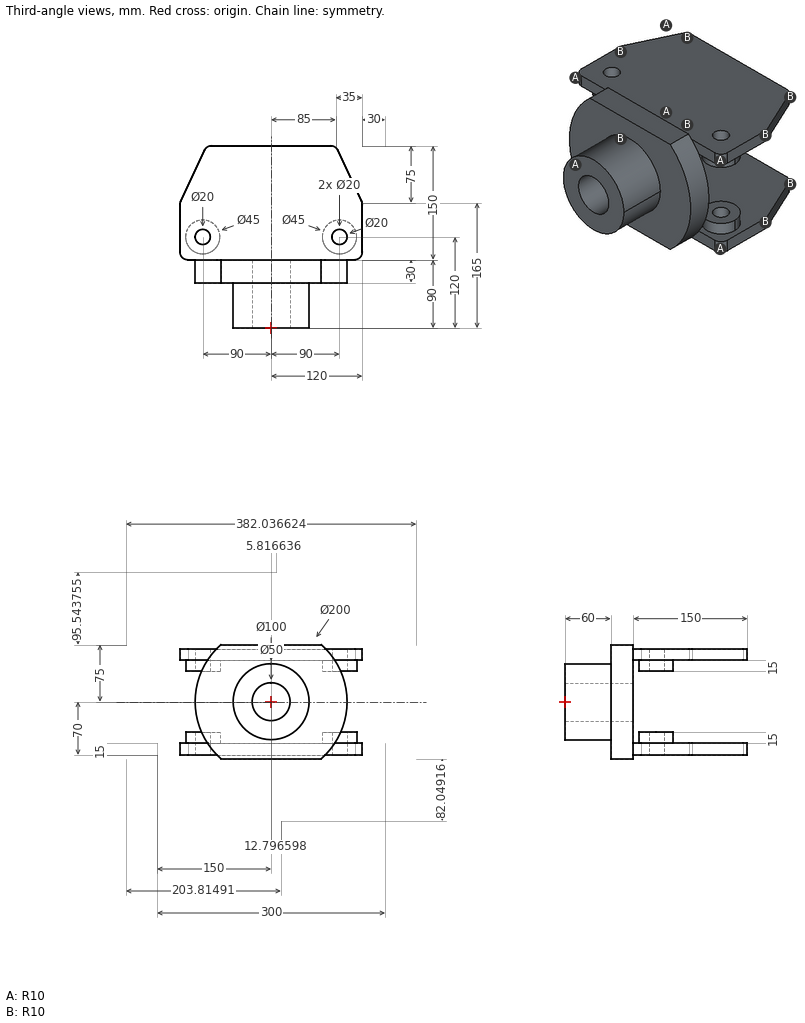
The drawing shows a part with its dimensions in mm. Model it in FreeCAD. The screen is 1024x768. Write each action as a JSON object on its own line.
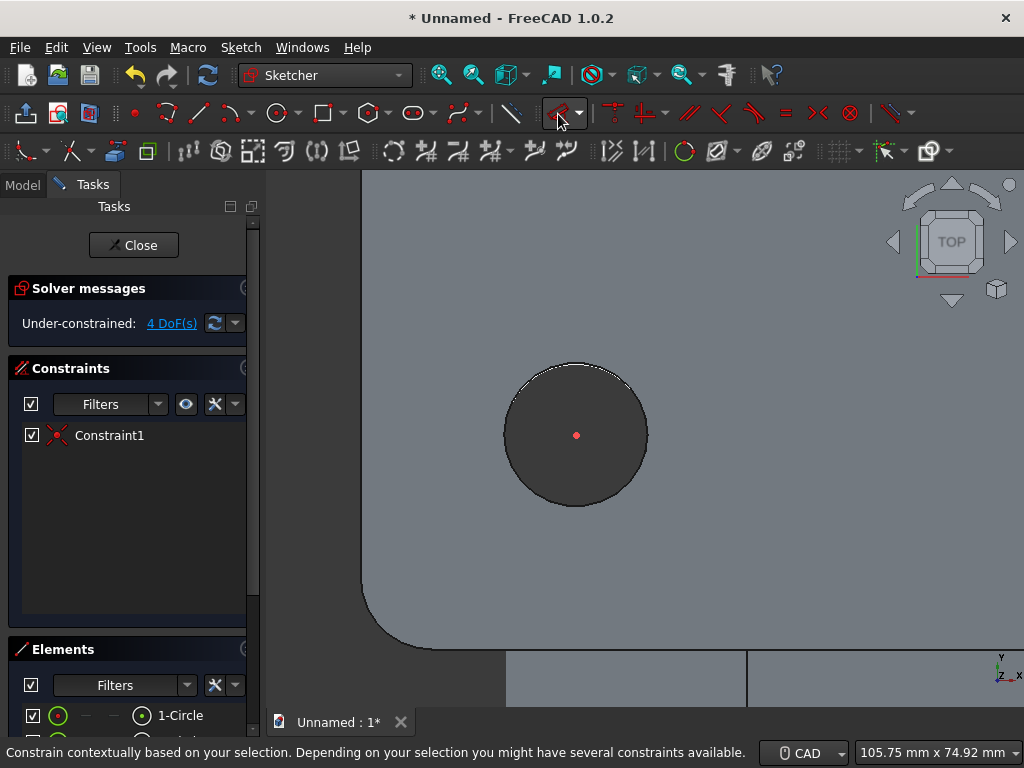
{"action": "left_click", "coordinate": [690, 322]}
{"action": "left_click", "coordinate": [713, 299]}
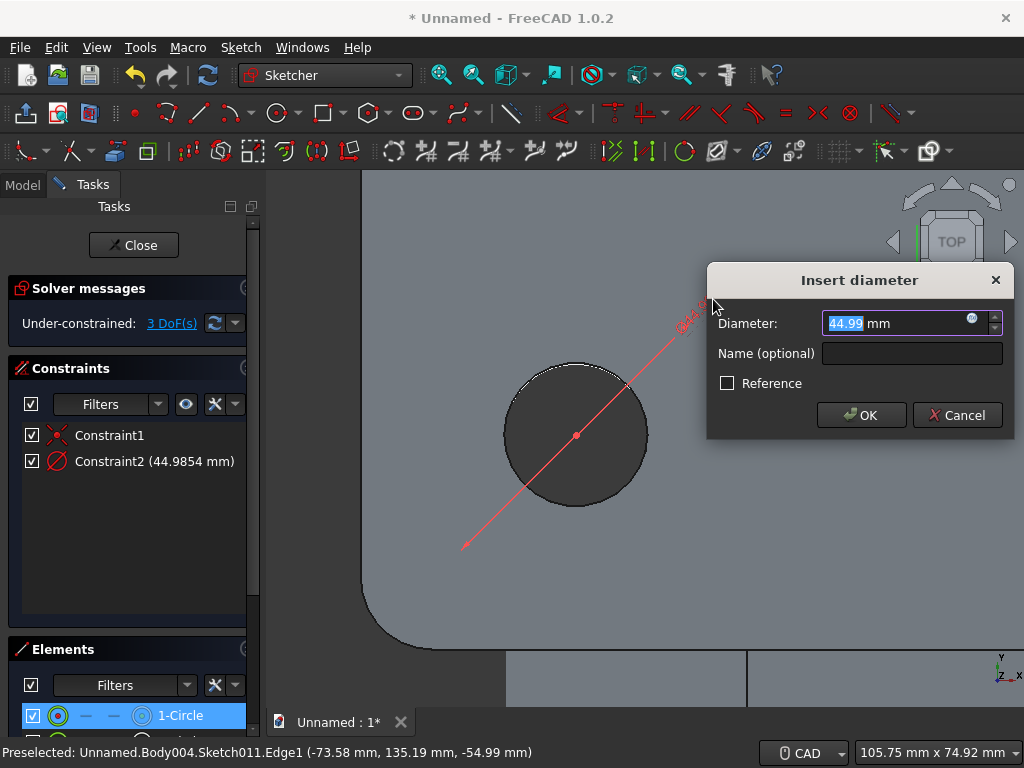
{"action": "type", "text": "45"}
{"action": "key", "text": "Return"}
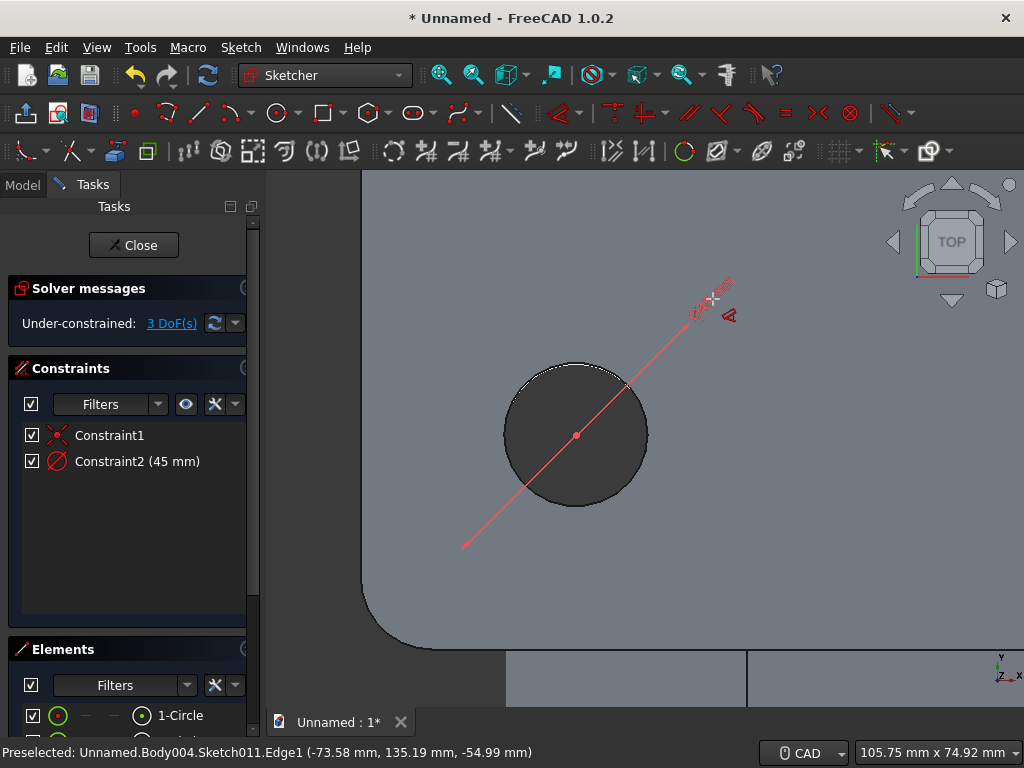
{"action": "left_click", "coordinate": [627, 385]}
{"action": "left_click", "coordinate": [650, 362]}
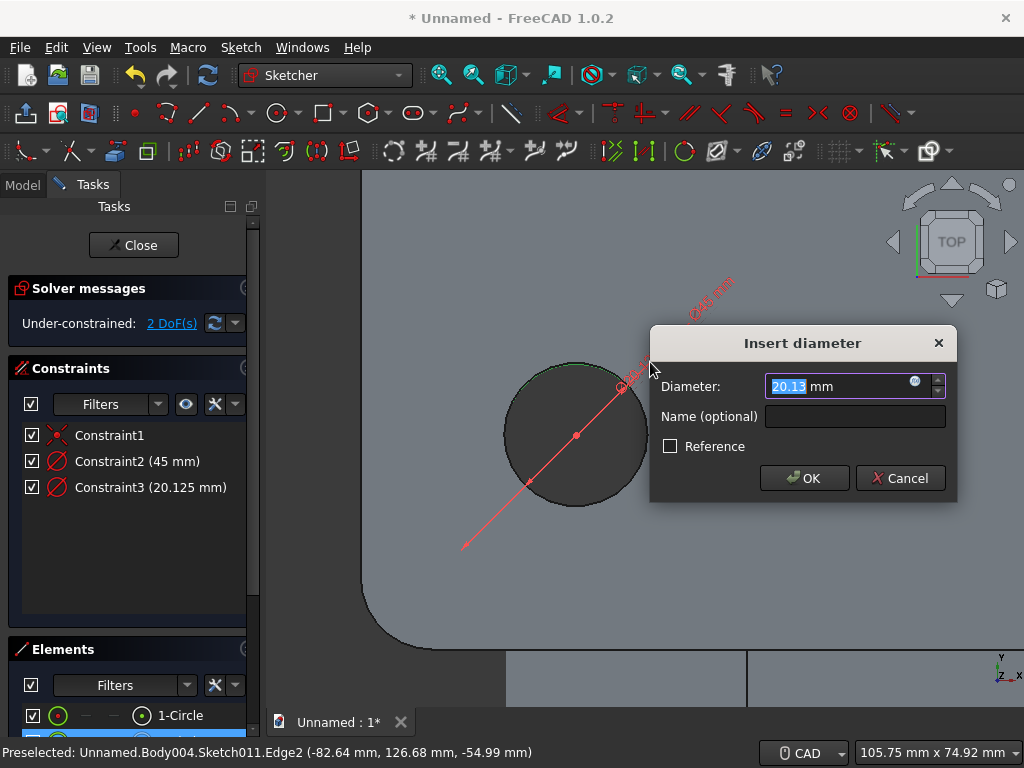
{"action": "type", "text": "20"}
{"action": "key", "text": "Return"}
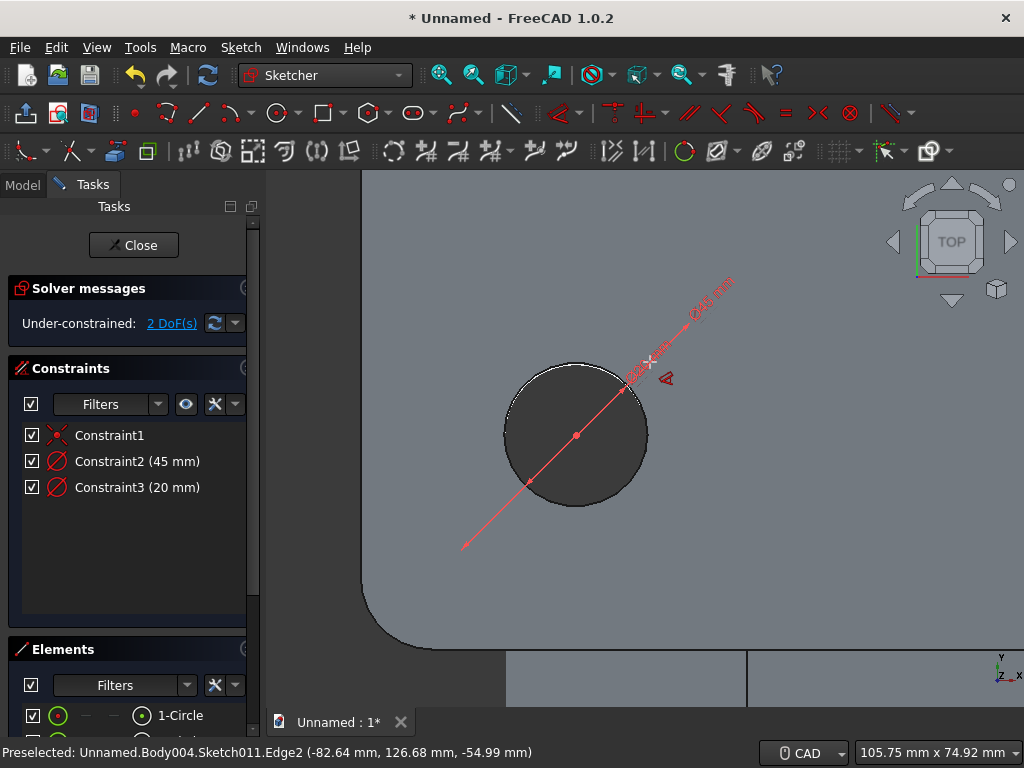
{"action": "left_click", "coordinate": [576, 436]}
{"action": "left_click", "coordinate": [718, 402]}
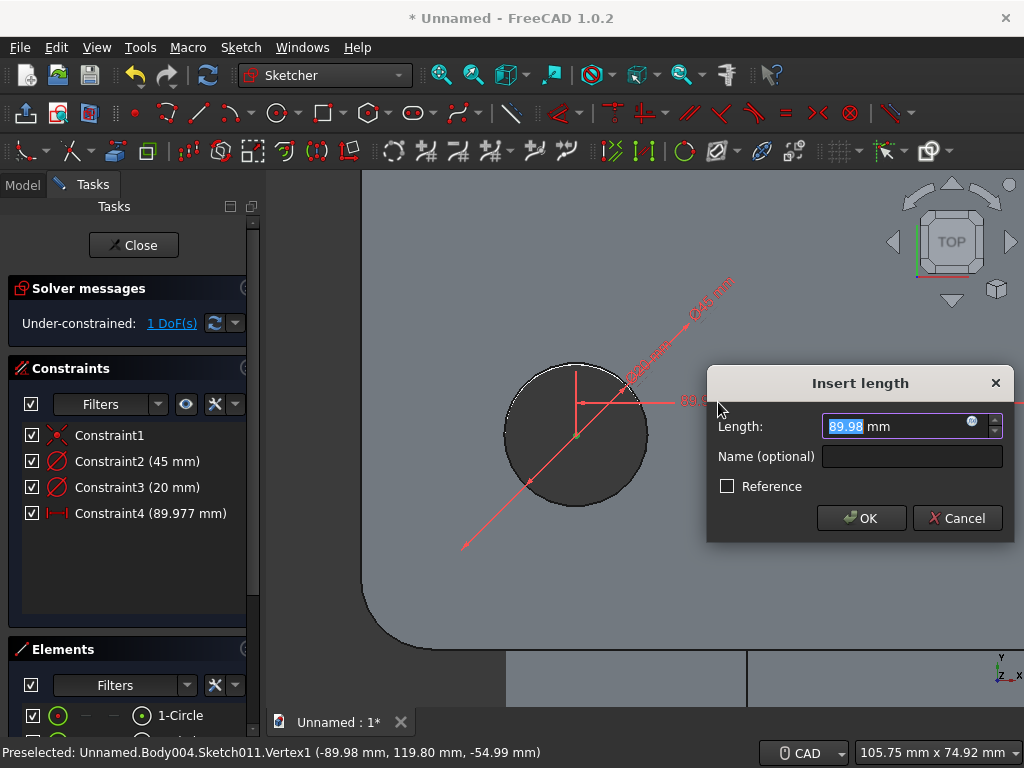
{"action": "type", "text": "90"}
{"action": "key", "text": "Return"}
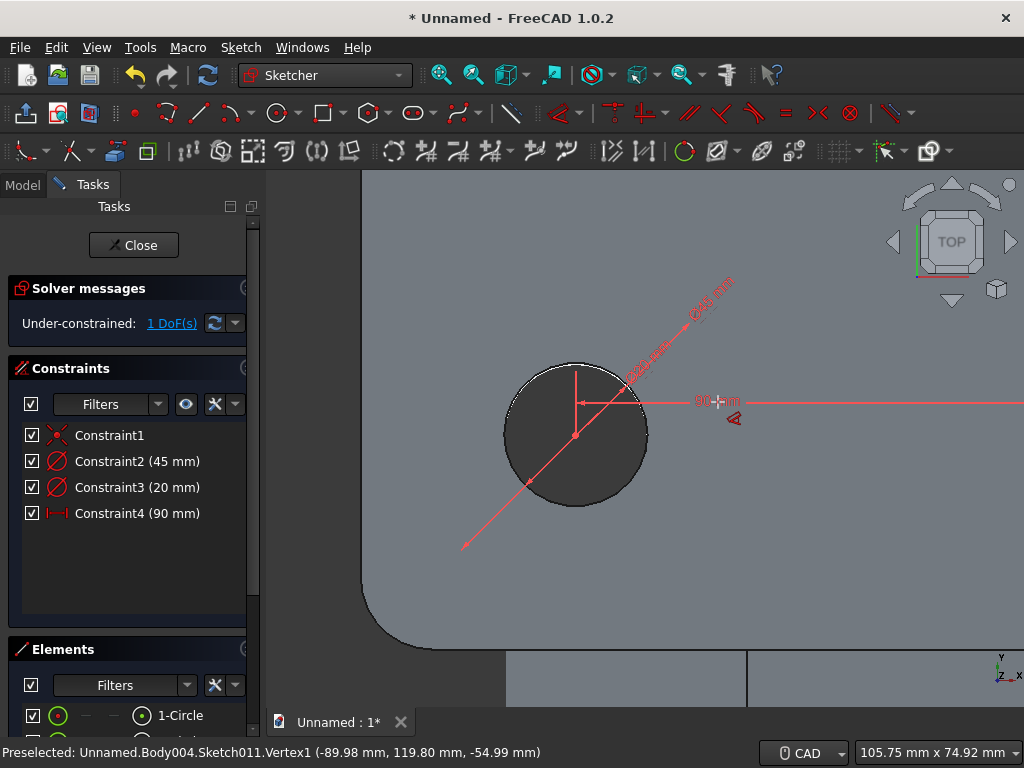
{"action": "left_click", "coordinate": [576, 436]}
{"action": "left_click", "coordinate": [542, 558]}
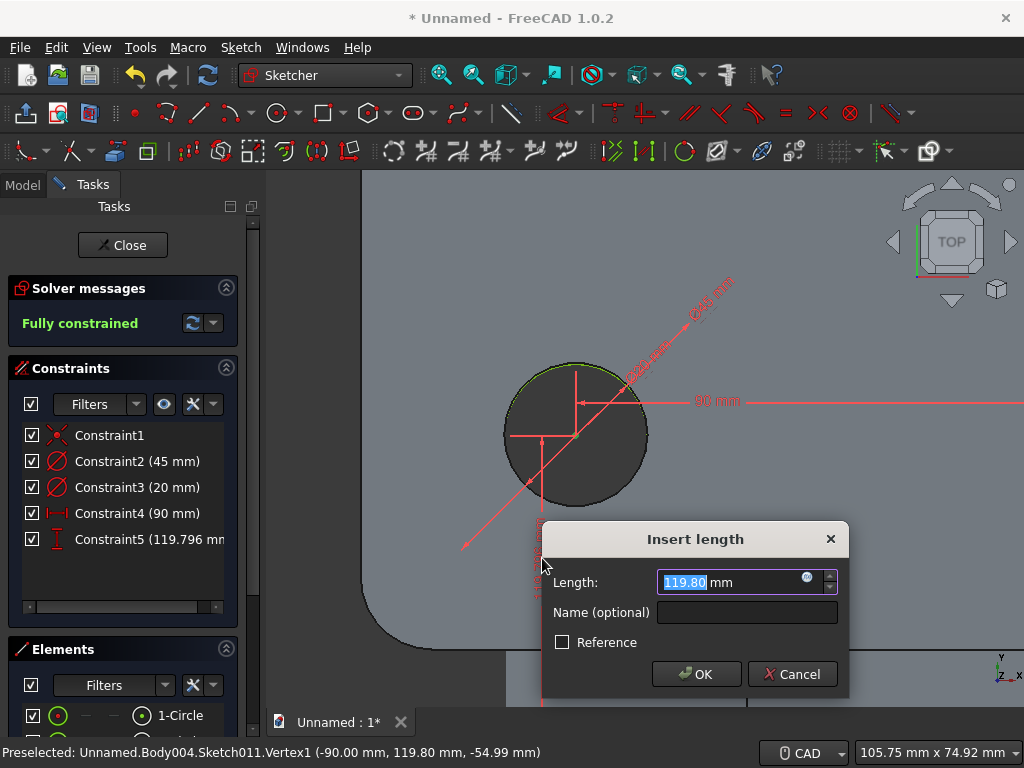
{"action": "type", "text": "120"}
{"action": "key", "text": "Return"}
{"action": "key", "text": "Escape"}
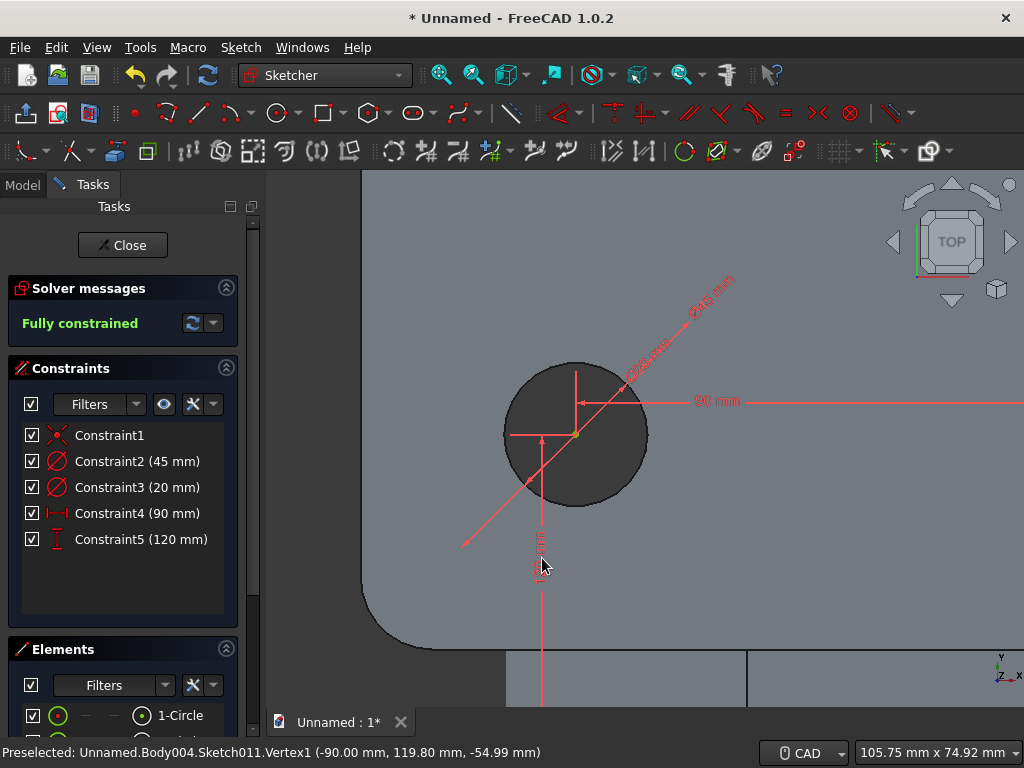
{"action": "left_click", "coordinate": [123, 245]}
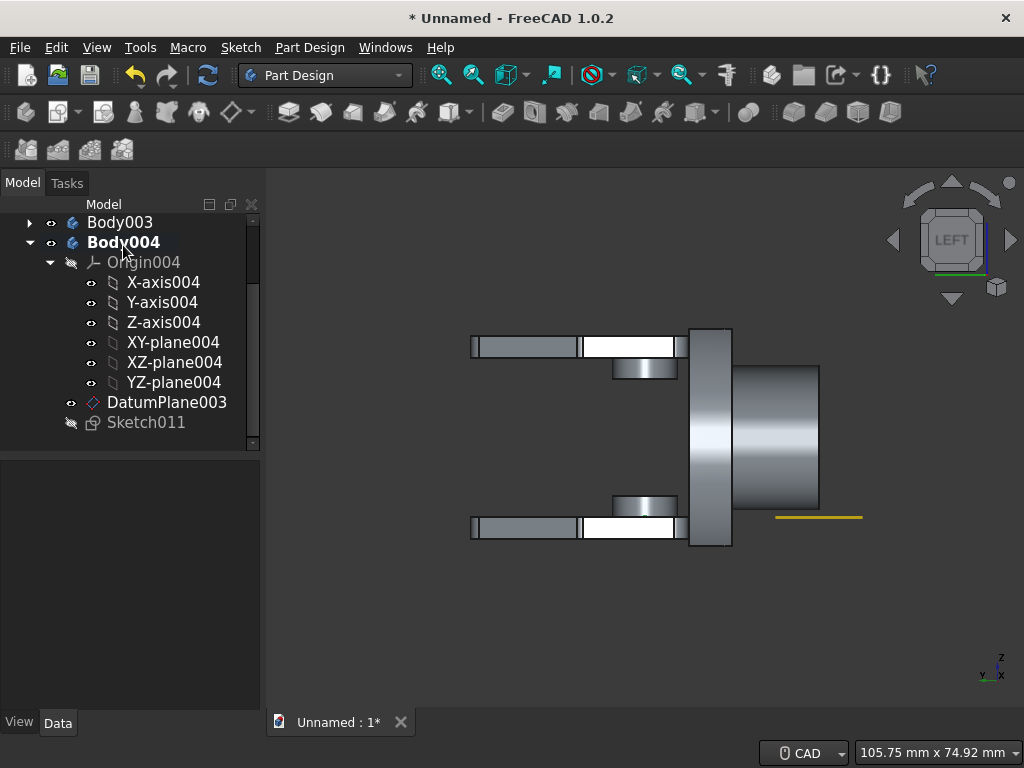
{"action": "left_click", "coordinate": [290, 112]}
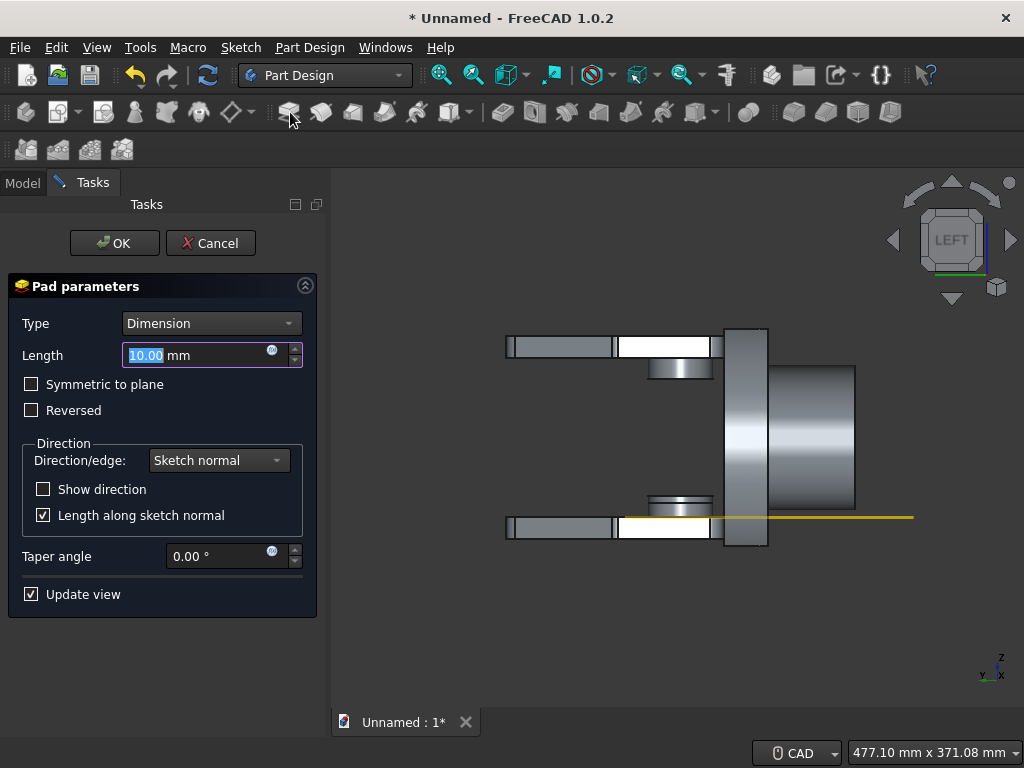
{"action": "type", "text": "15"}
{"action": "key", "text": "Tab"}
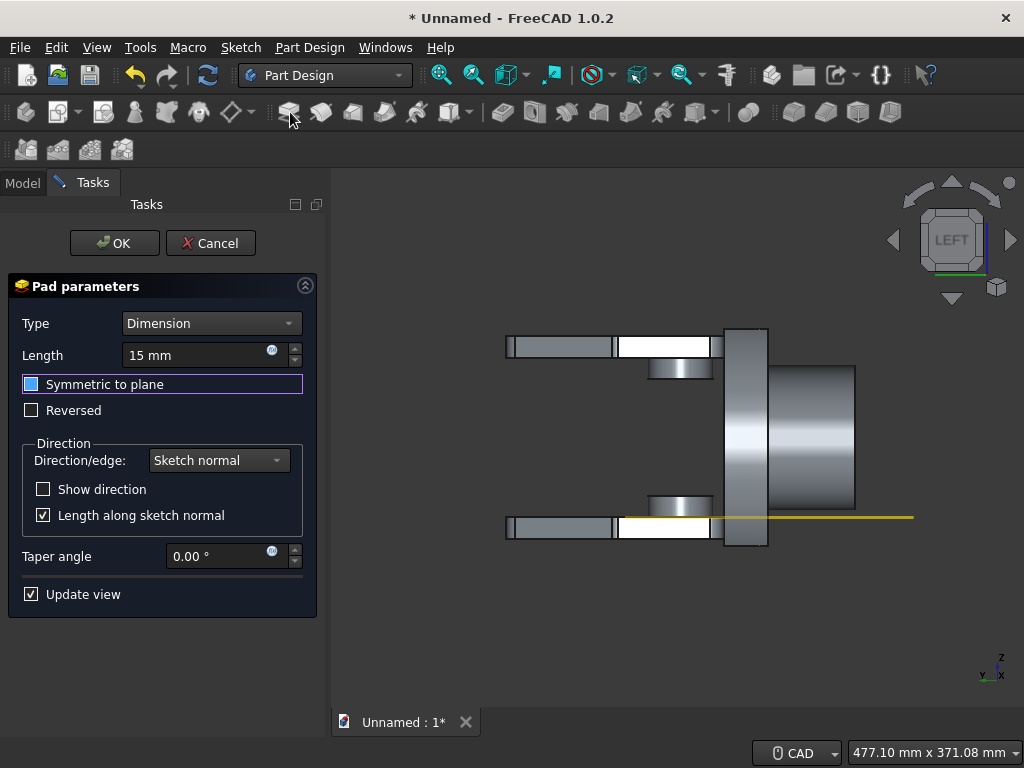
{"action": "left_click", "coordinate": [115, 243]}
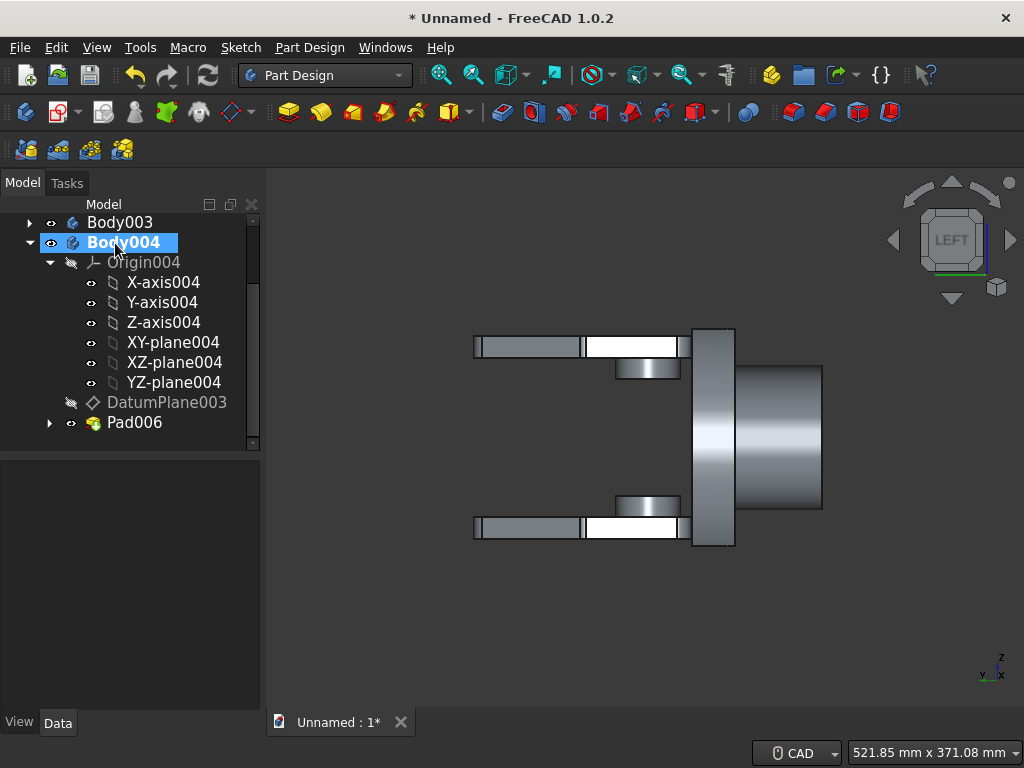
{"action": "key", "text": "0"}